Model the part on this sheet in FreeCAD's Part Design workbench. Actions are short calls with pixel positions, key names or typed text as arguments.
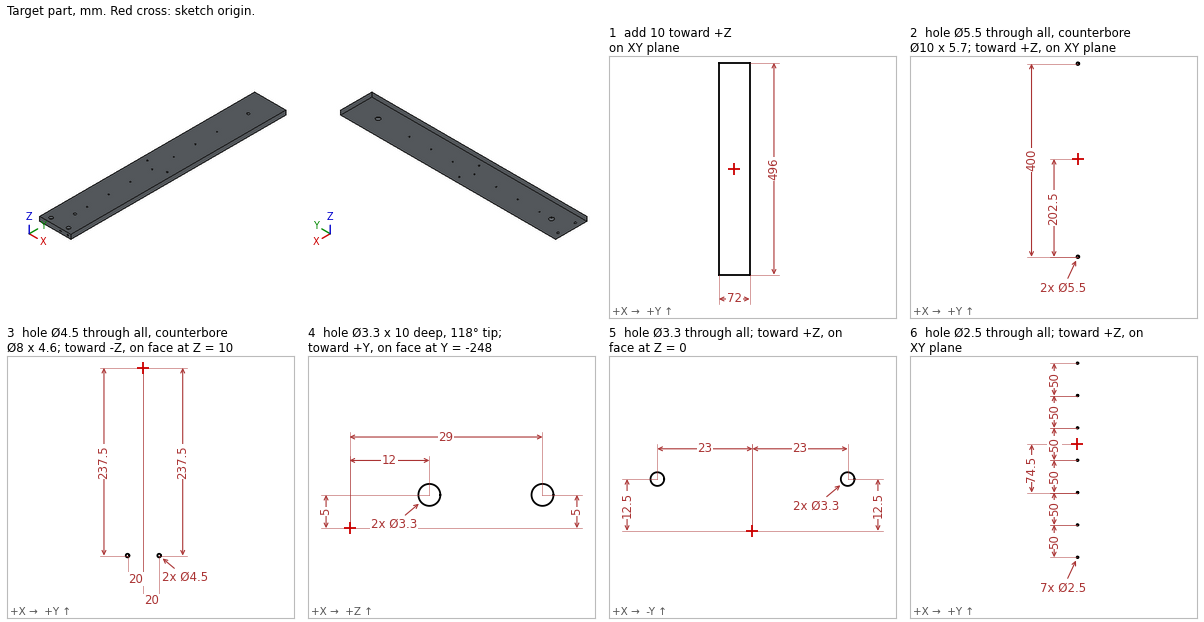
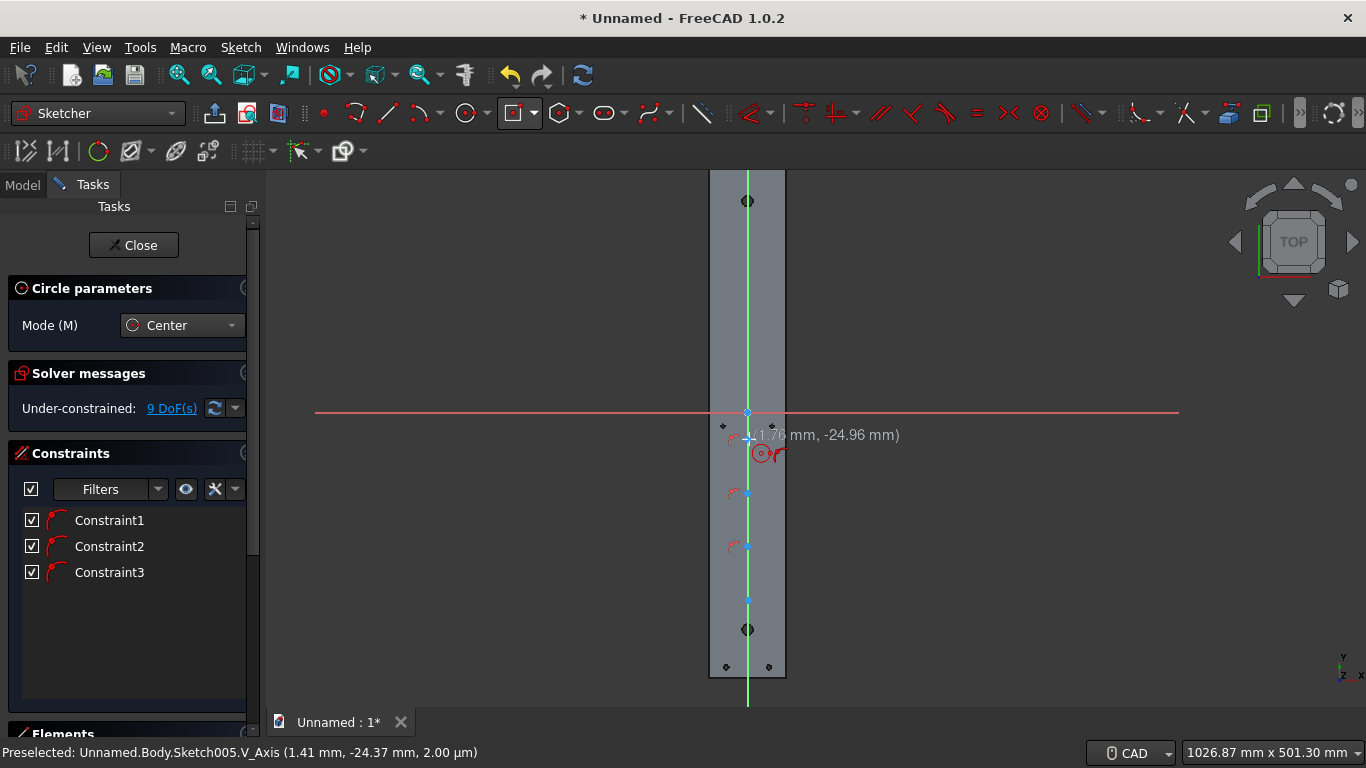
scroll(748, 385, up, 15)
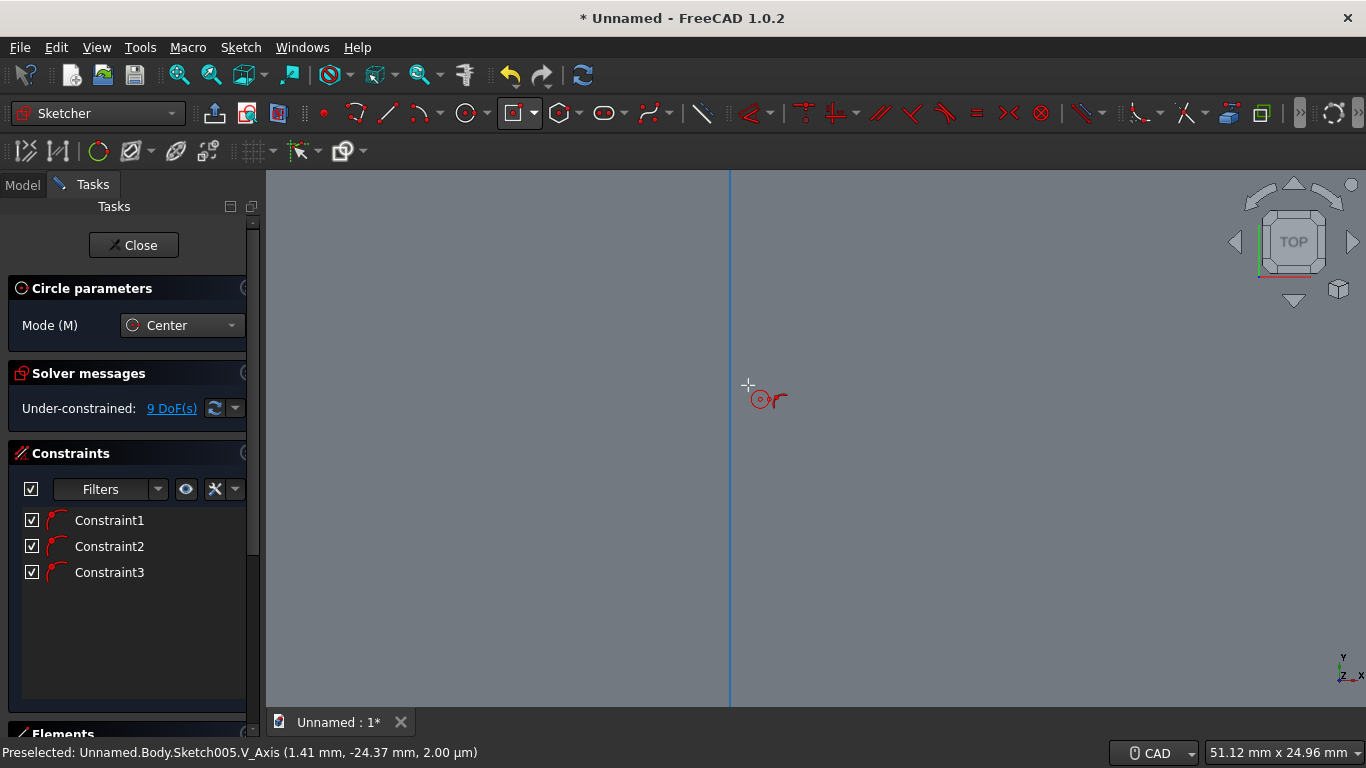
scroll(748, 385, down, 15)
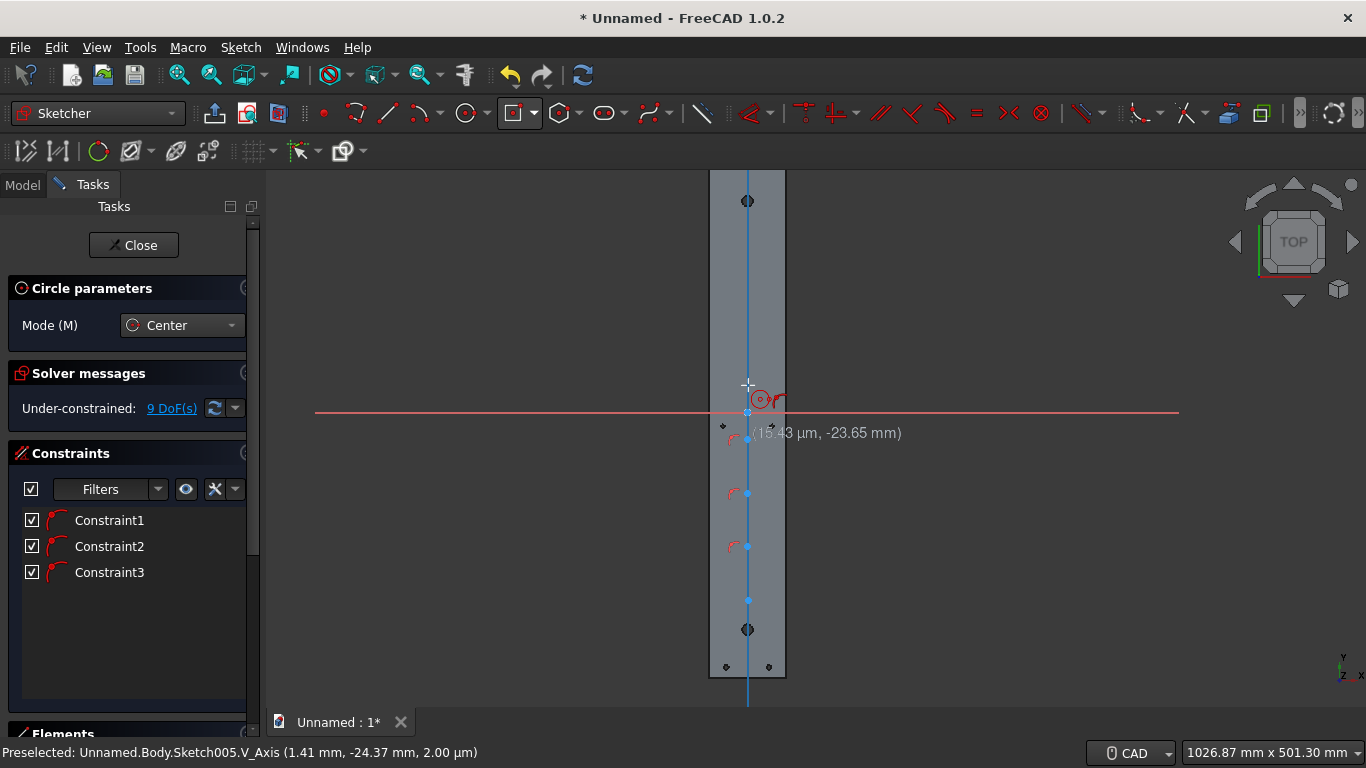
click(748, 385)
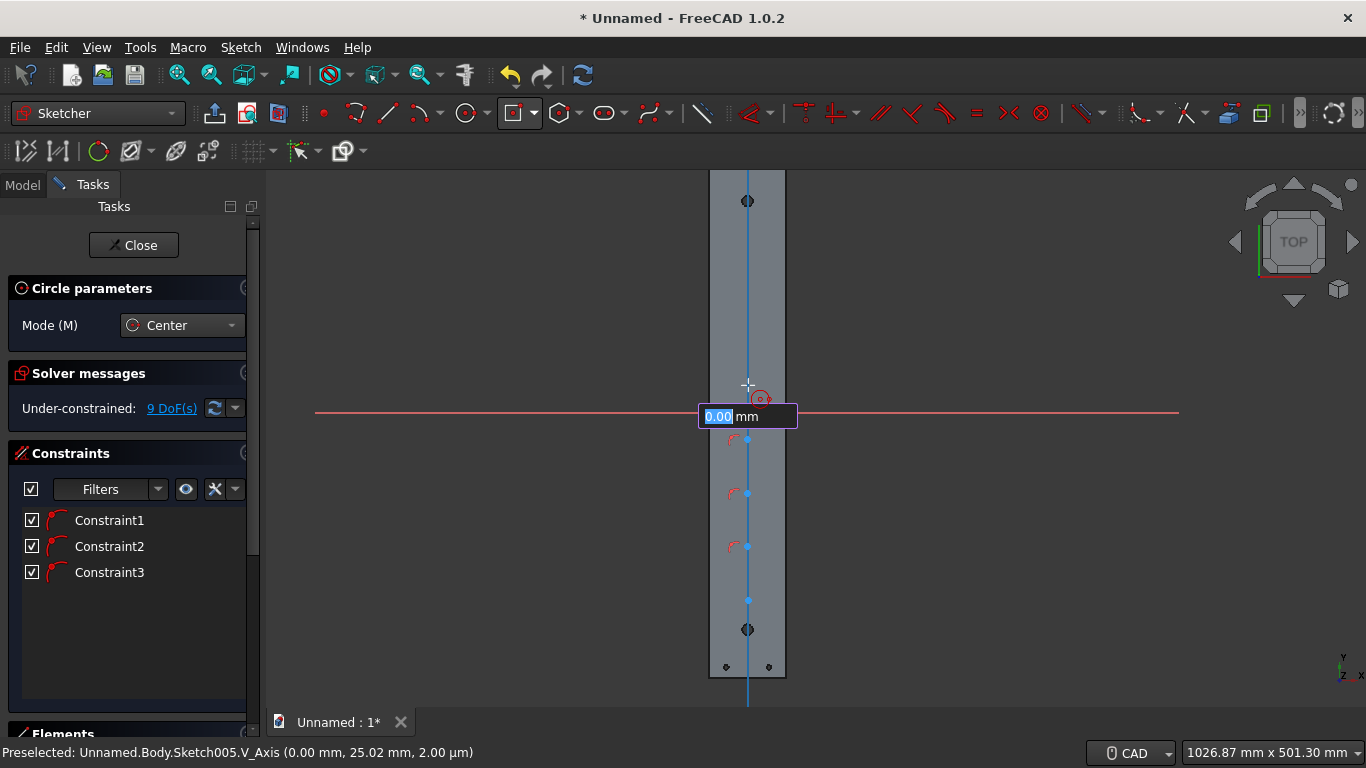
scroll(749, 385, up, 13)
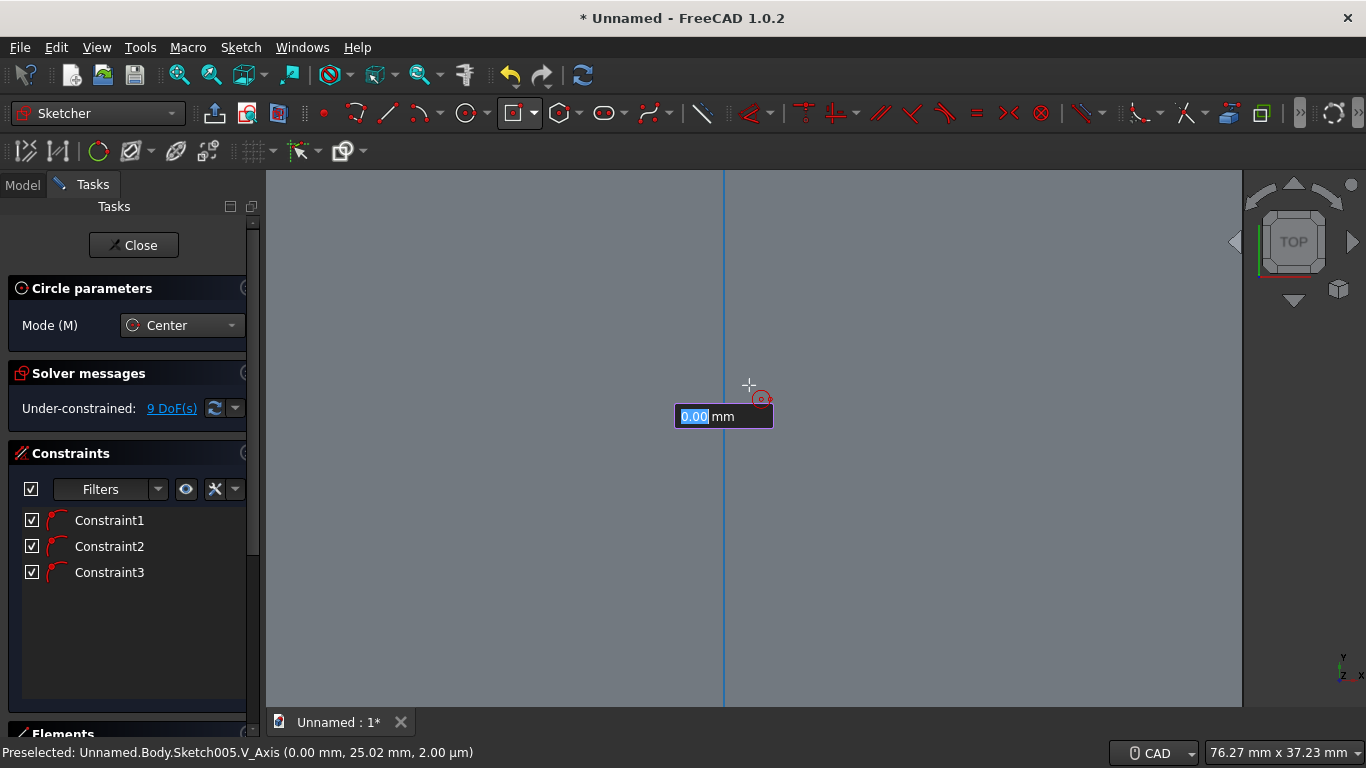
click(741, 380)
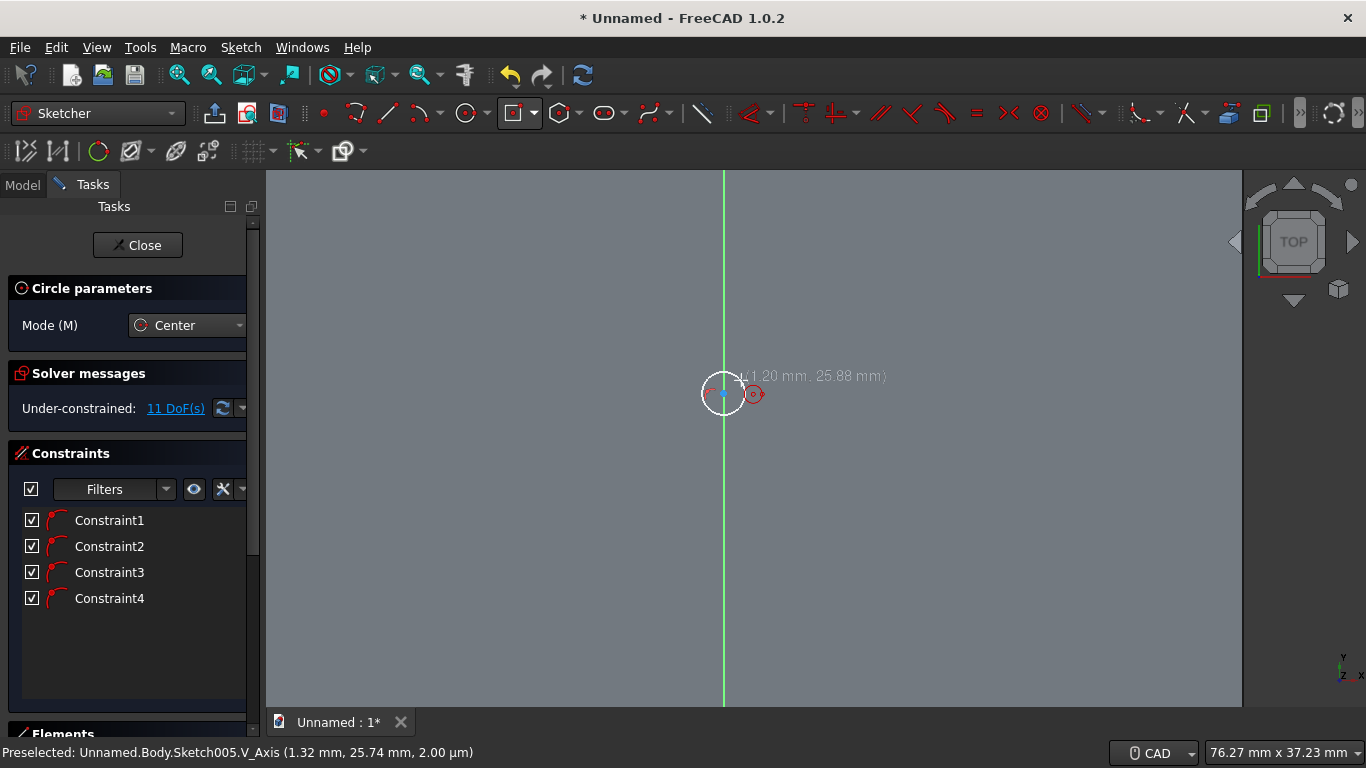
scroll(749, 385, down, 13)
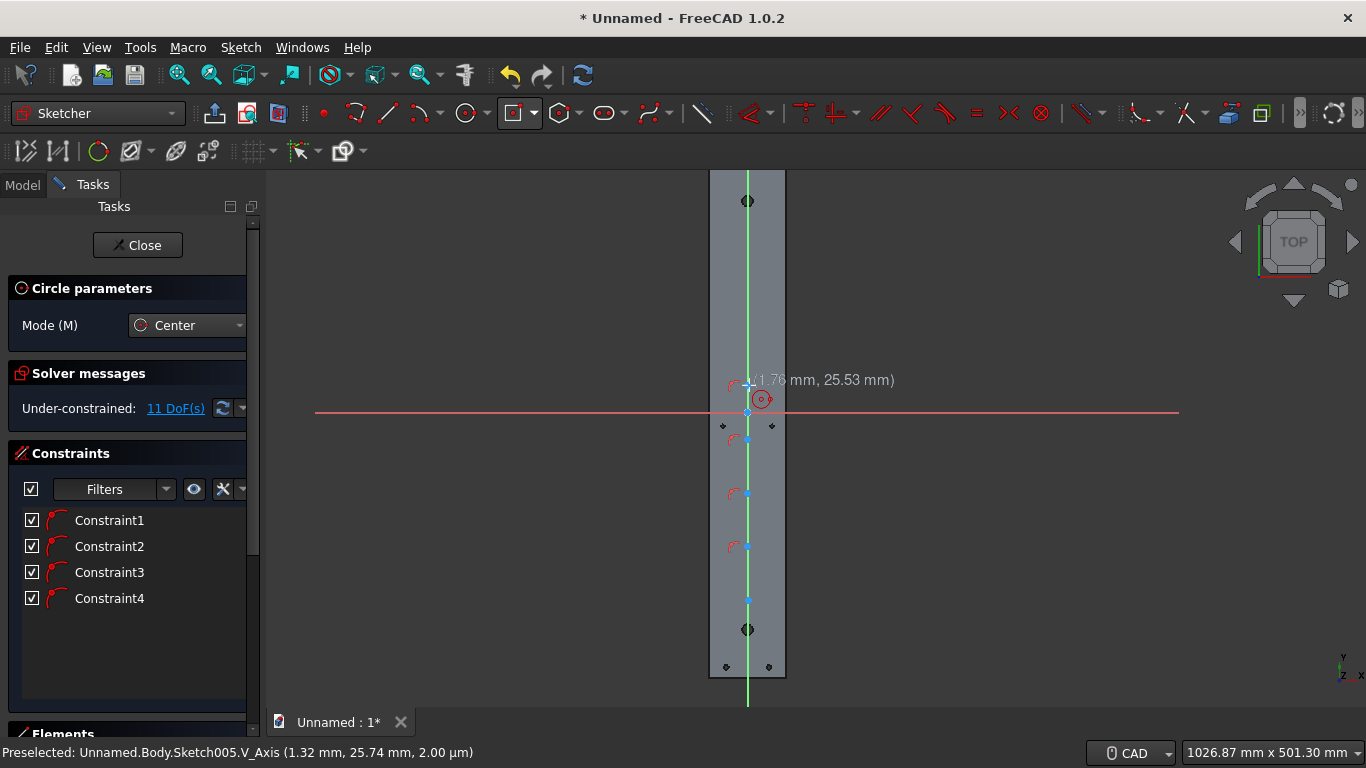
scroll(748, 332, up, 15)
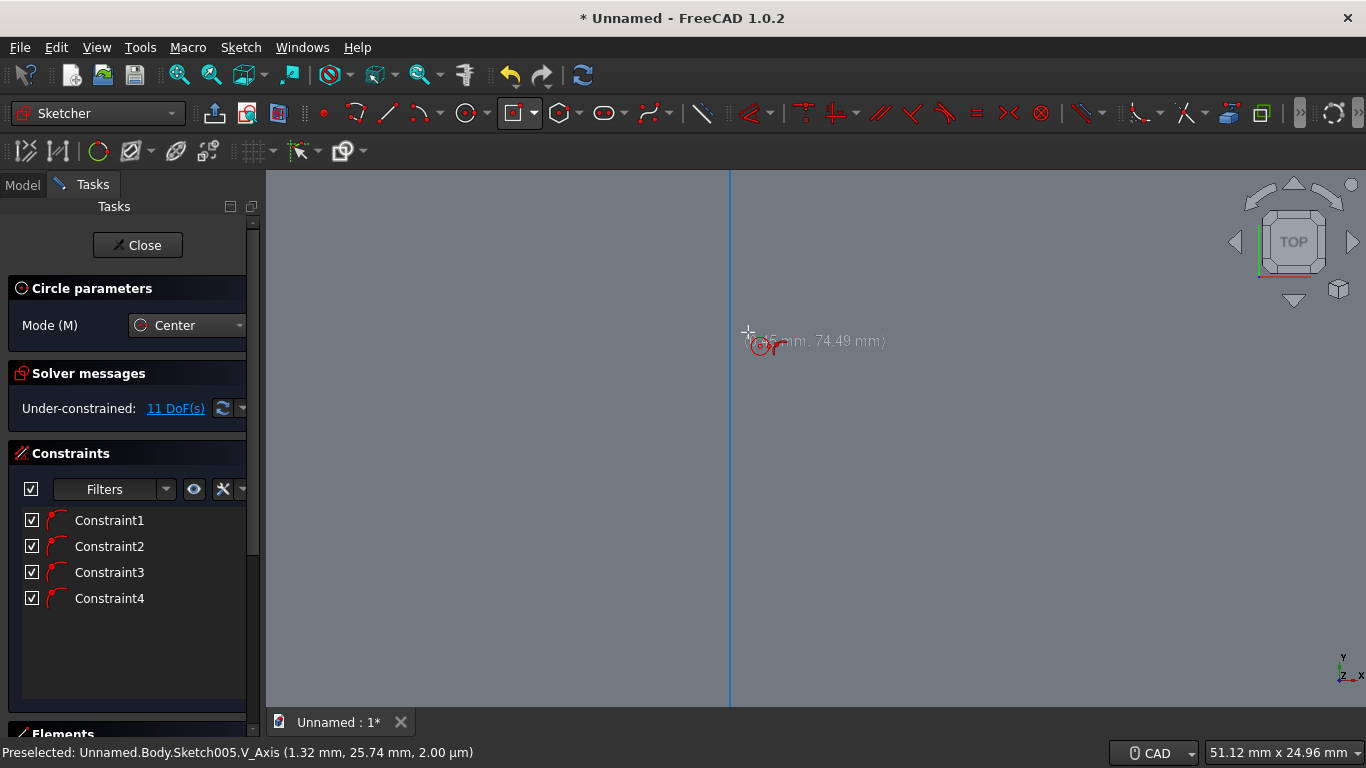
scroll(748, 332, down, 15)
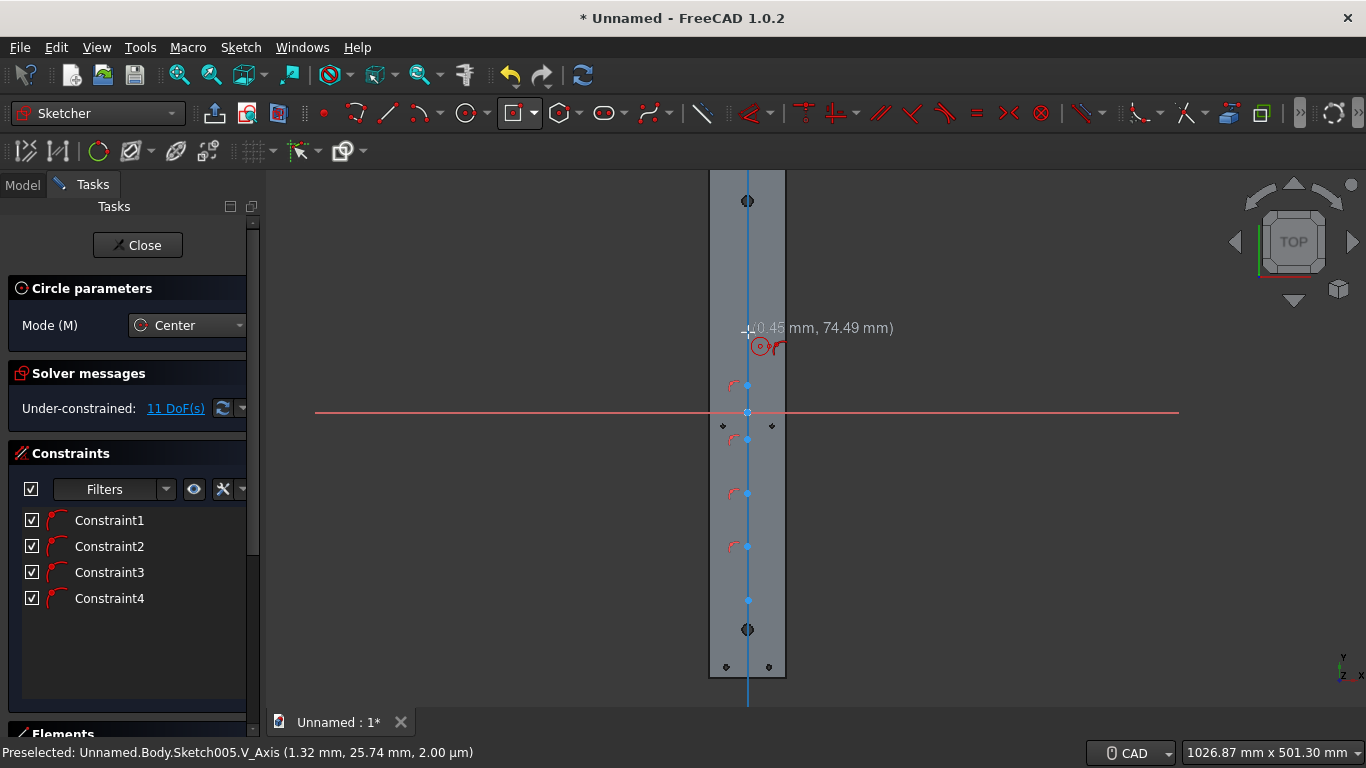
click(748, 332)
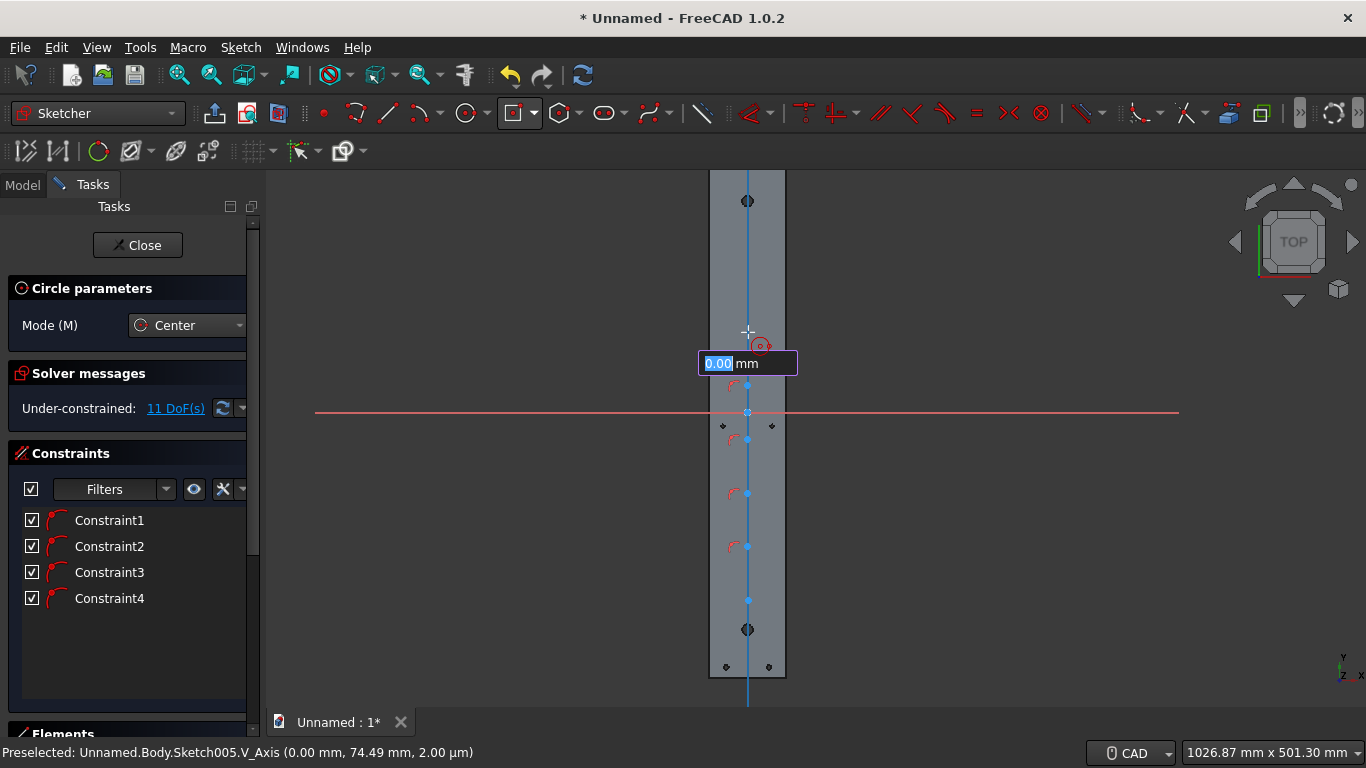
scroll(749, 331, up, 13)